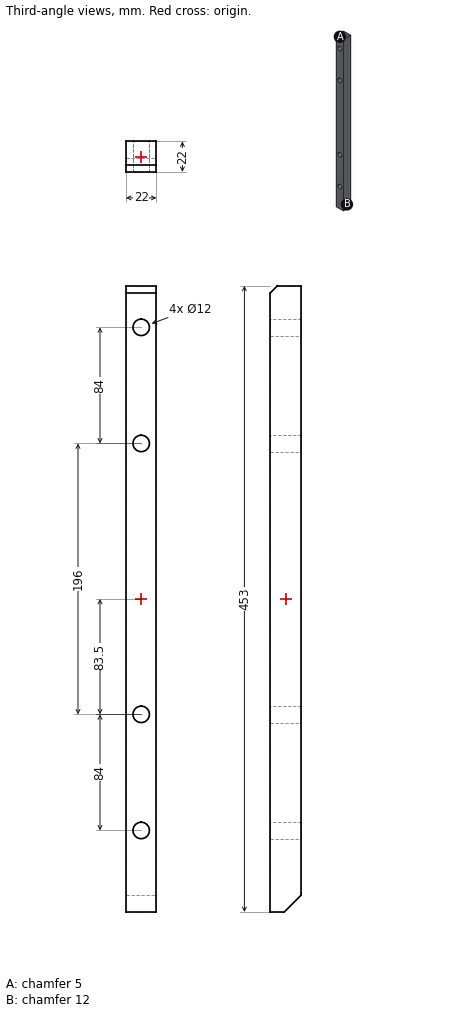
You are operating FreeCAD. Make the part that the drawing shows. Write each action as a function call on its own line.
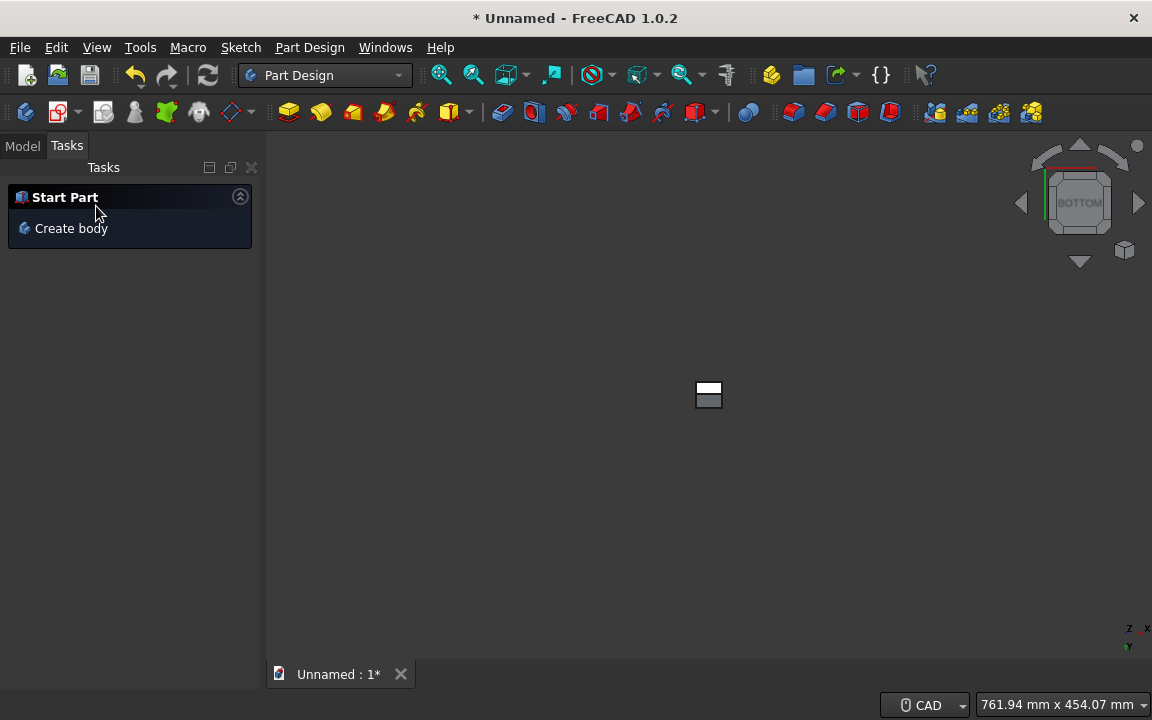
key(0)